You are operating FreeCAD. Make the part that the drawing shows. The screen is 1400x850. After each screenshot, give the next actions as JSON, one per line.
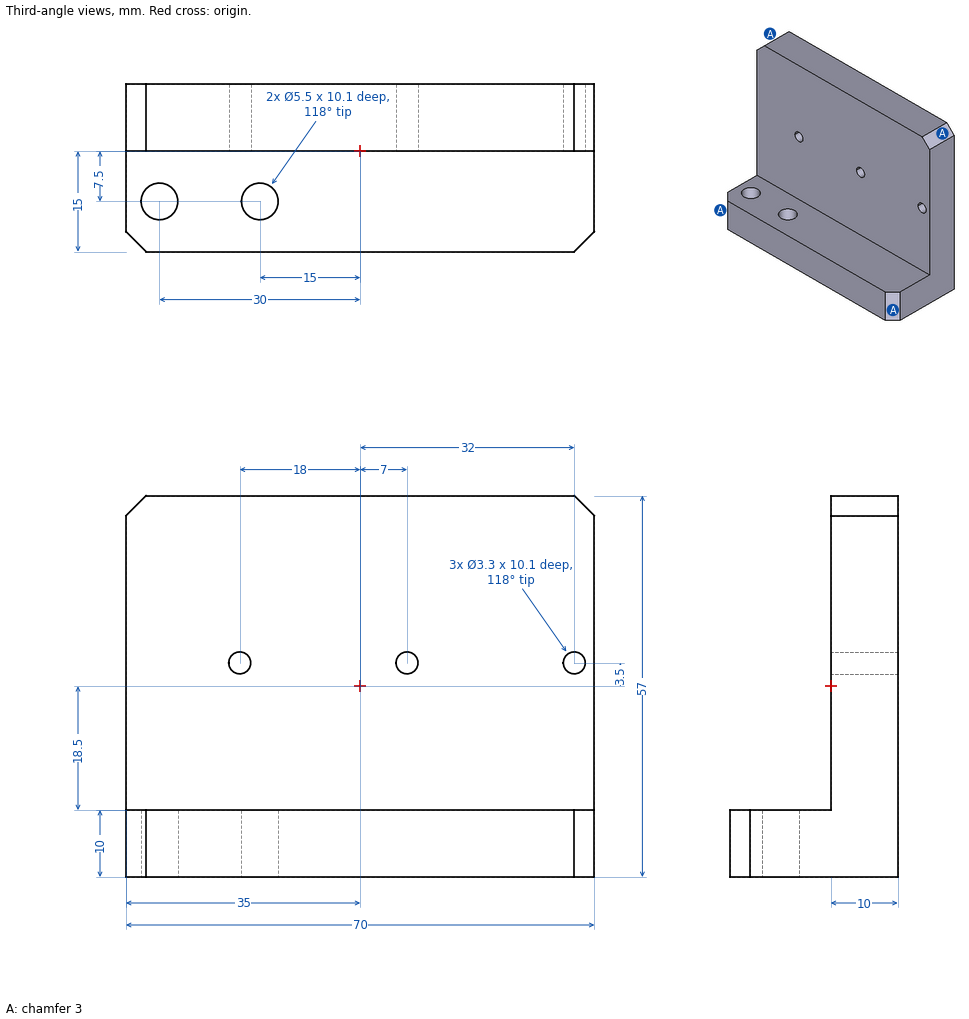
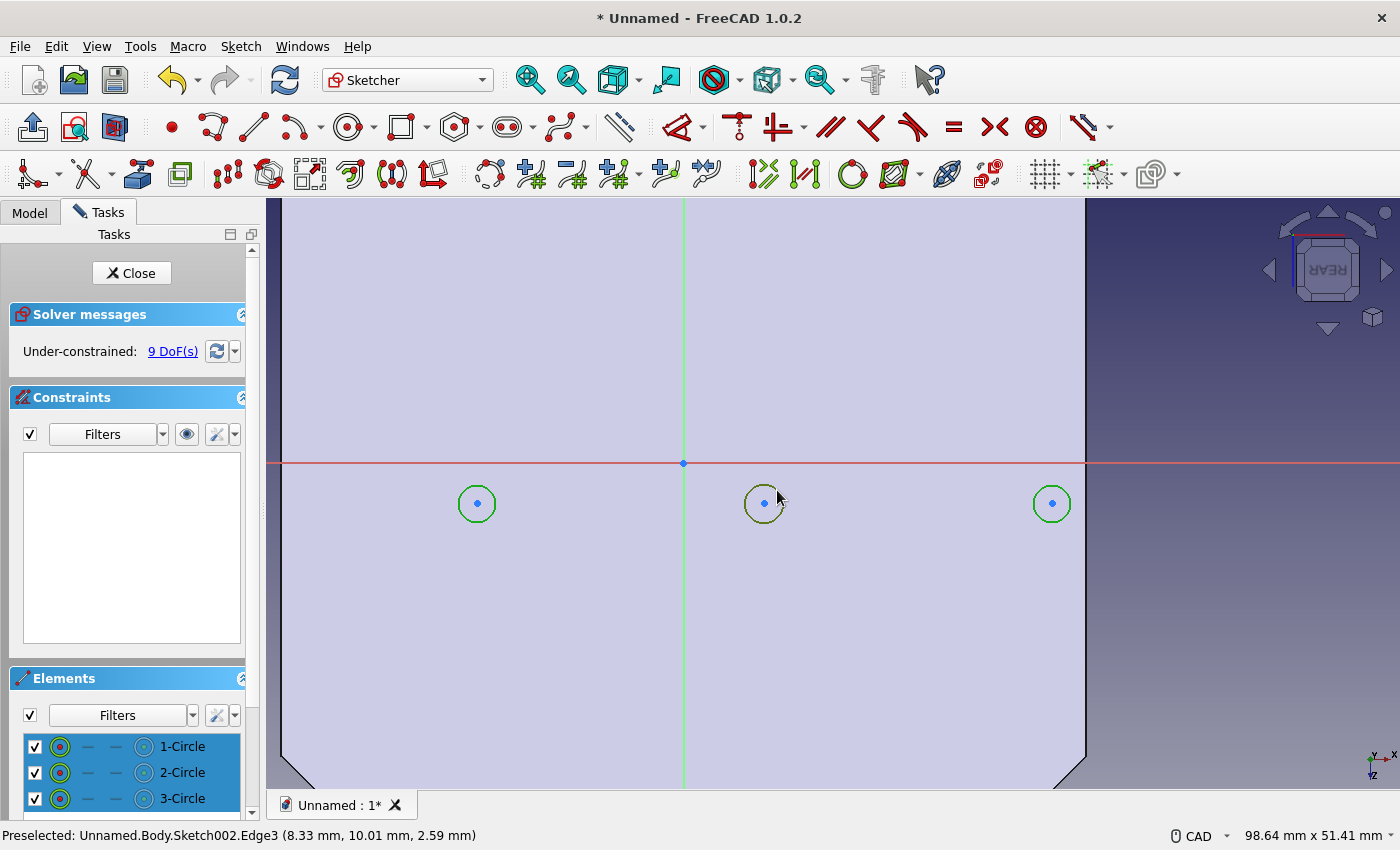
{"action": "left_click", "coordinate": [954, 128]}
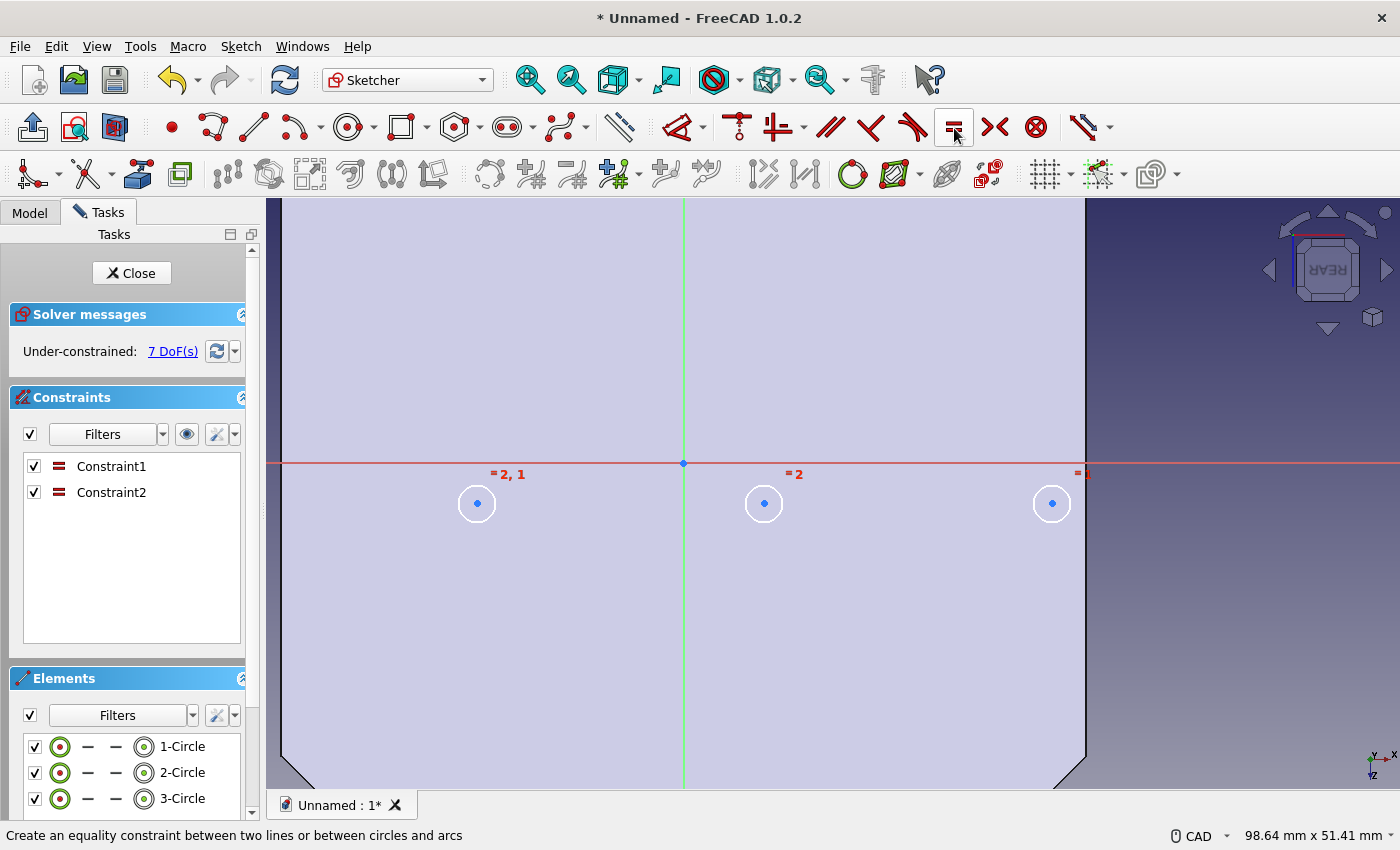
{"action": "left_click", "coordinate": [1052, 504]}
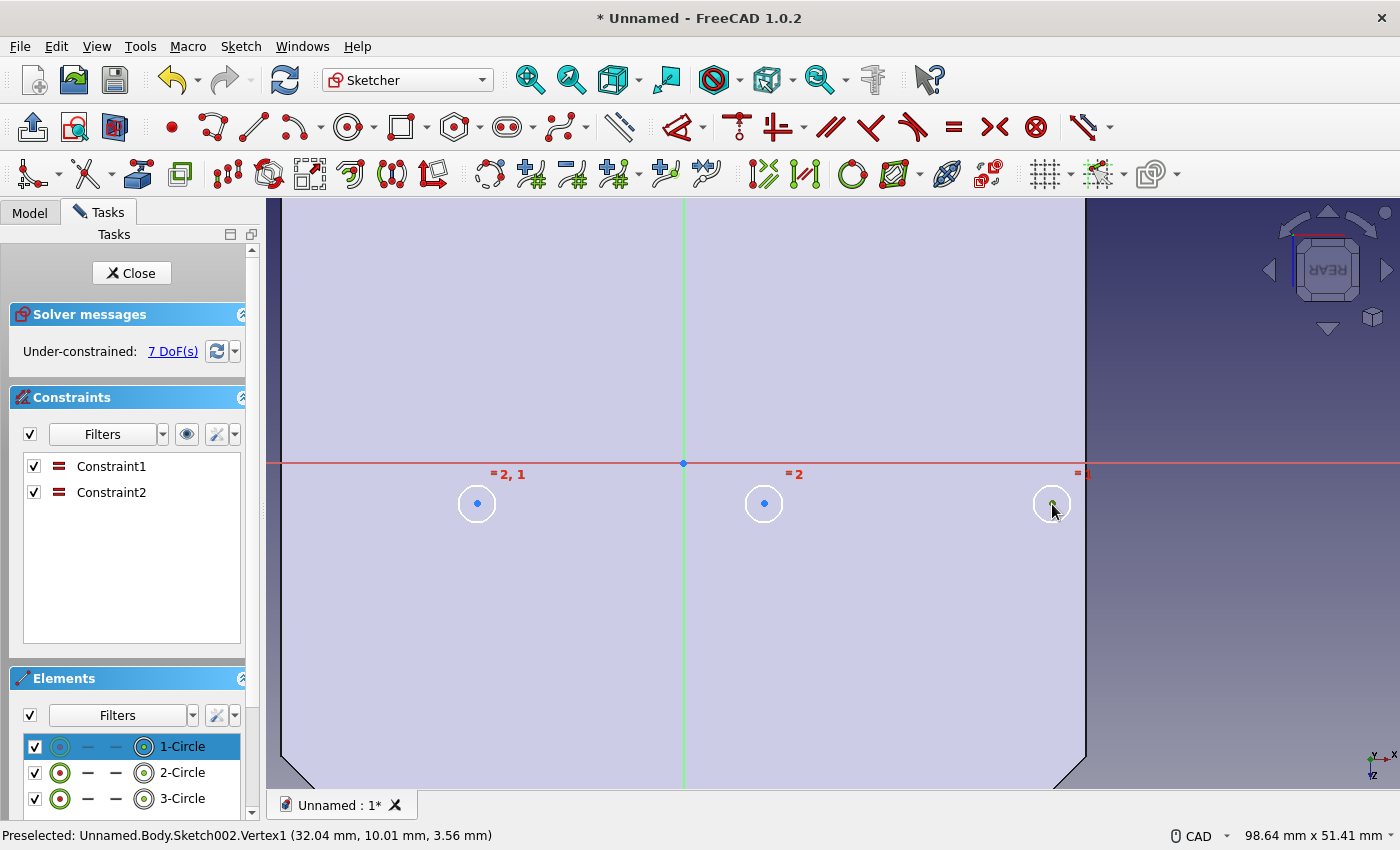
{"action": "left_click", "coordinate": [477, 504]}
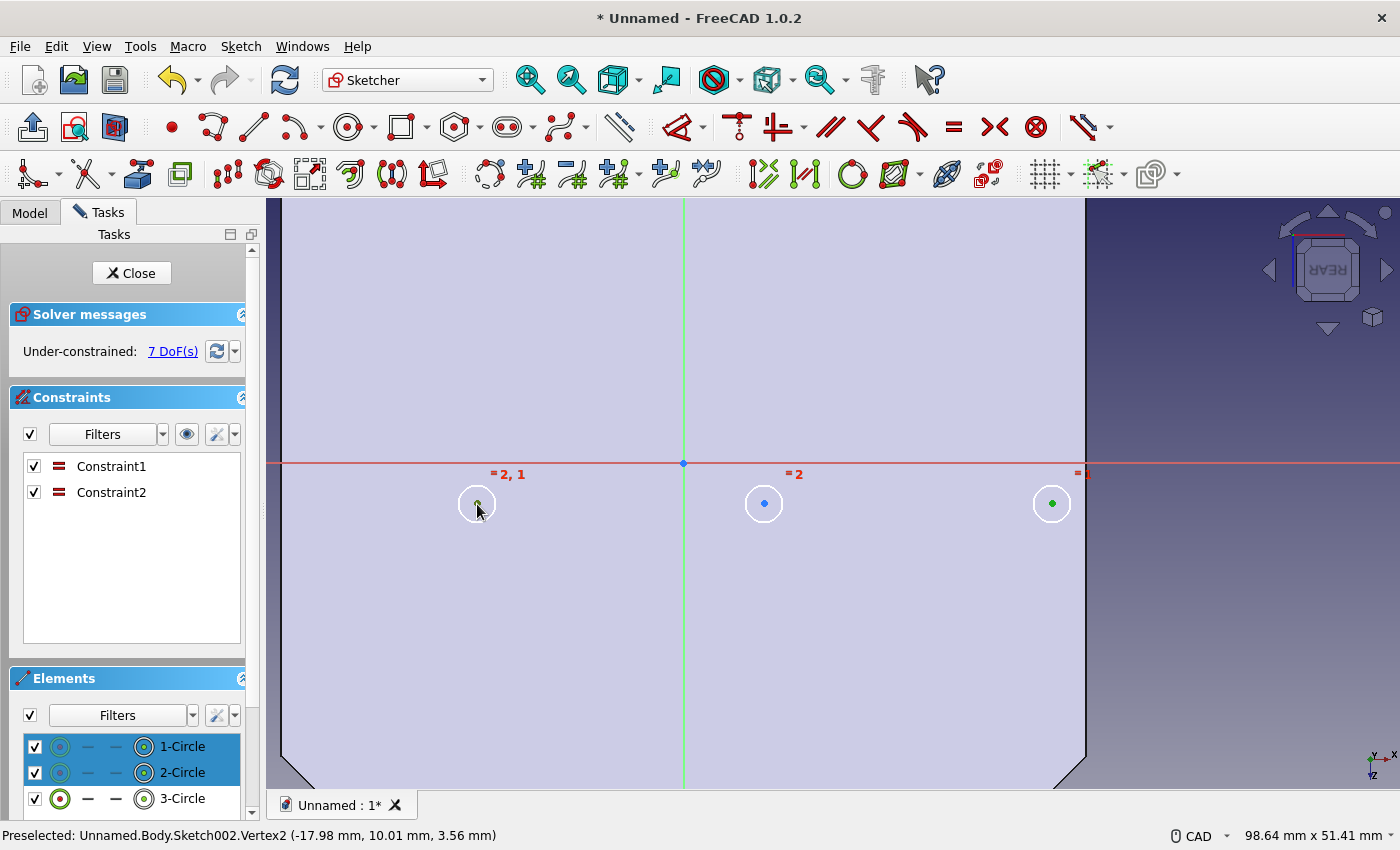
{"action": "left_click", "coordinate": [804, 128]}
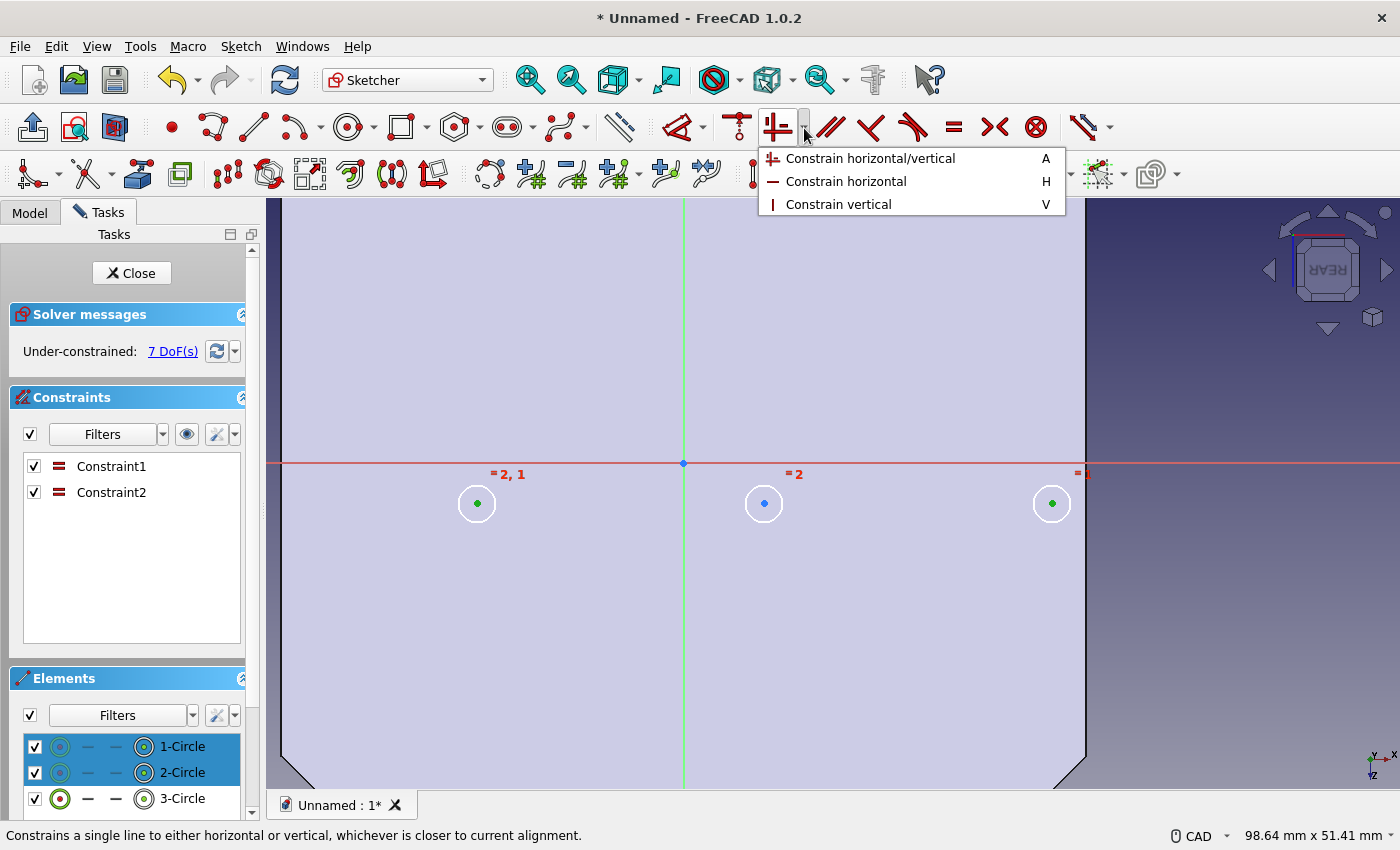
{"action": "left_click", "coordinate": [912, 182]}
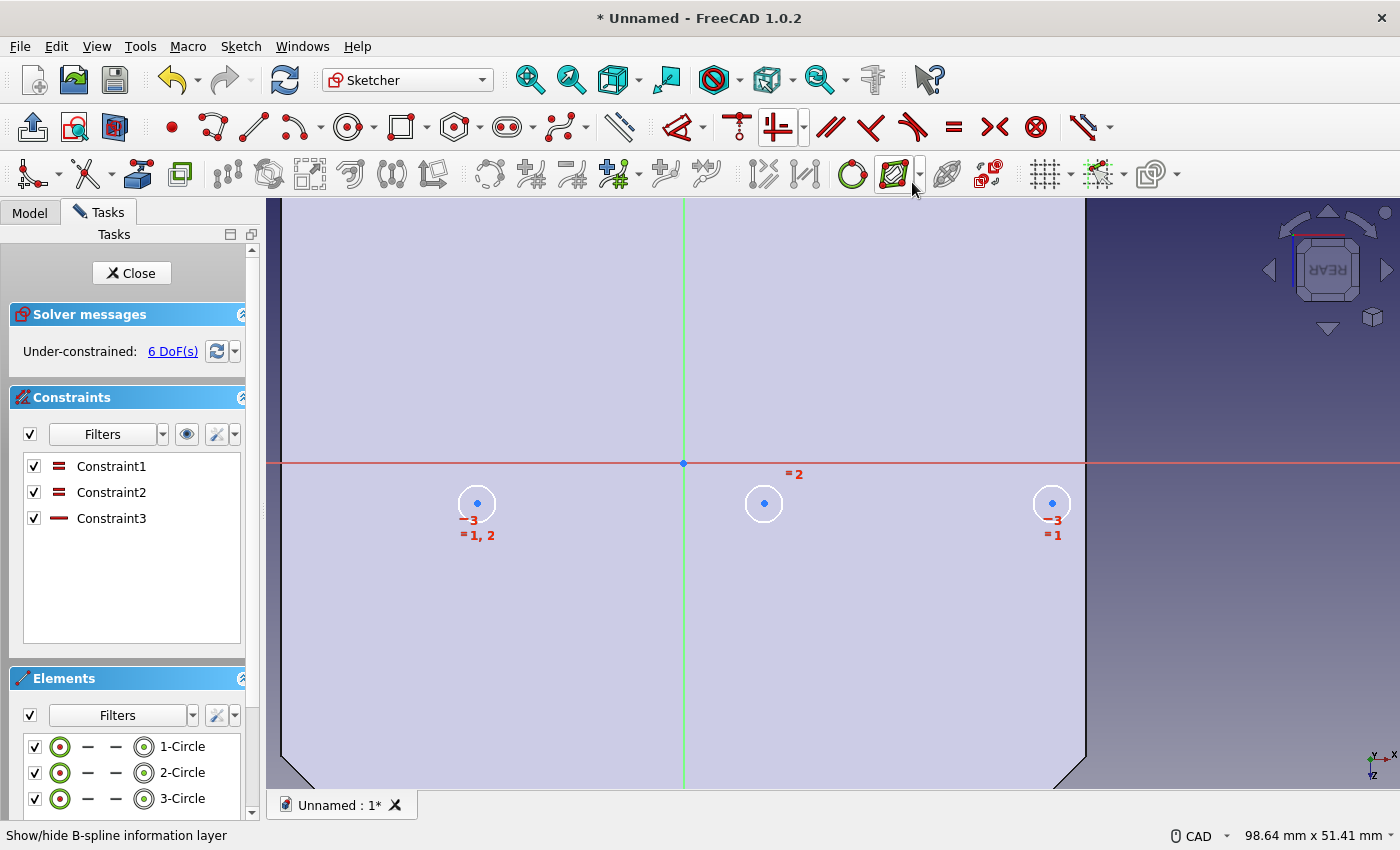
{"action": "left_click", "coordinate": [1052, 504]}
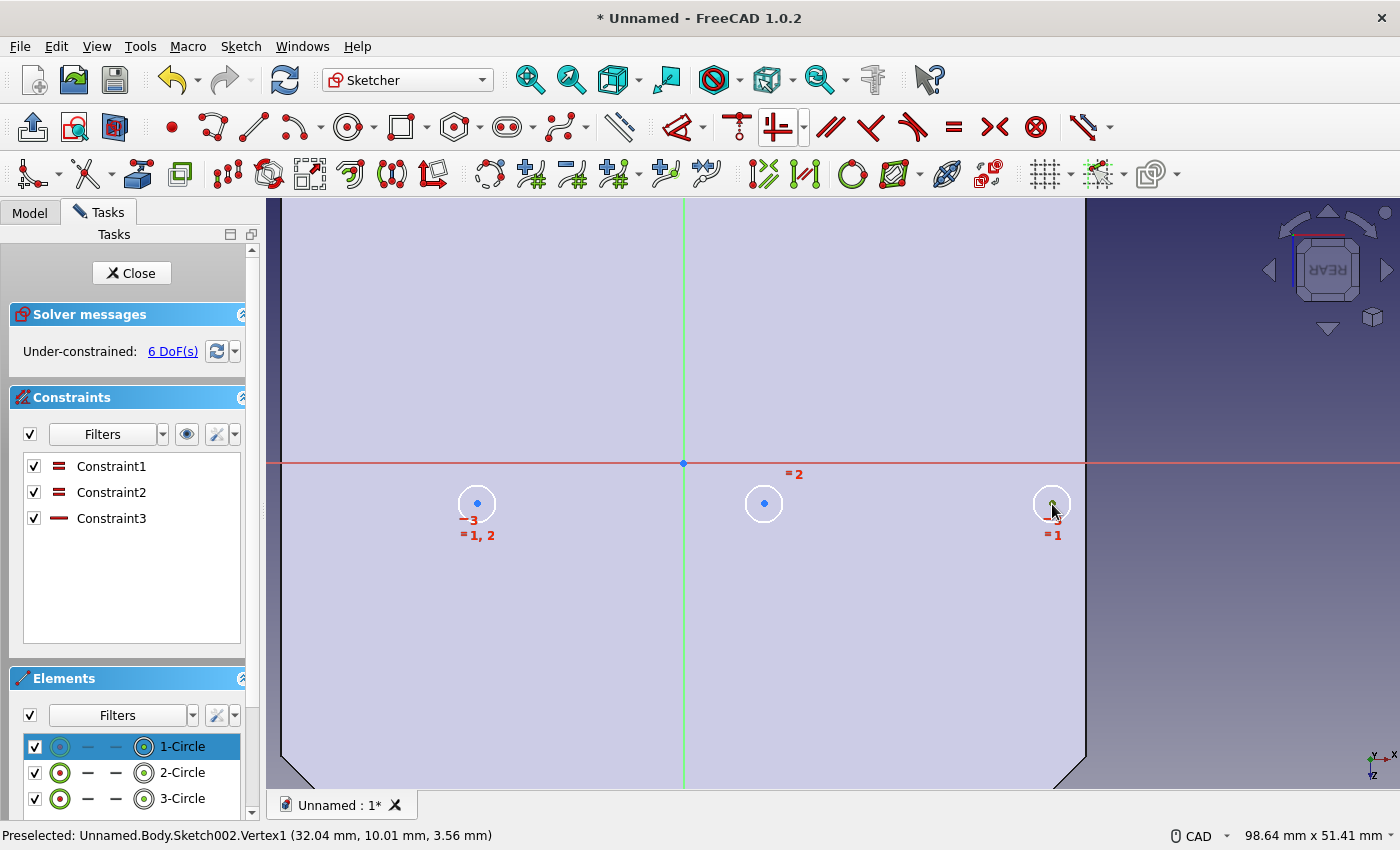
{"action": "left_click", "coordinate": [764, 504]}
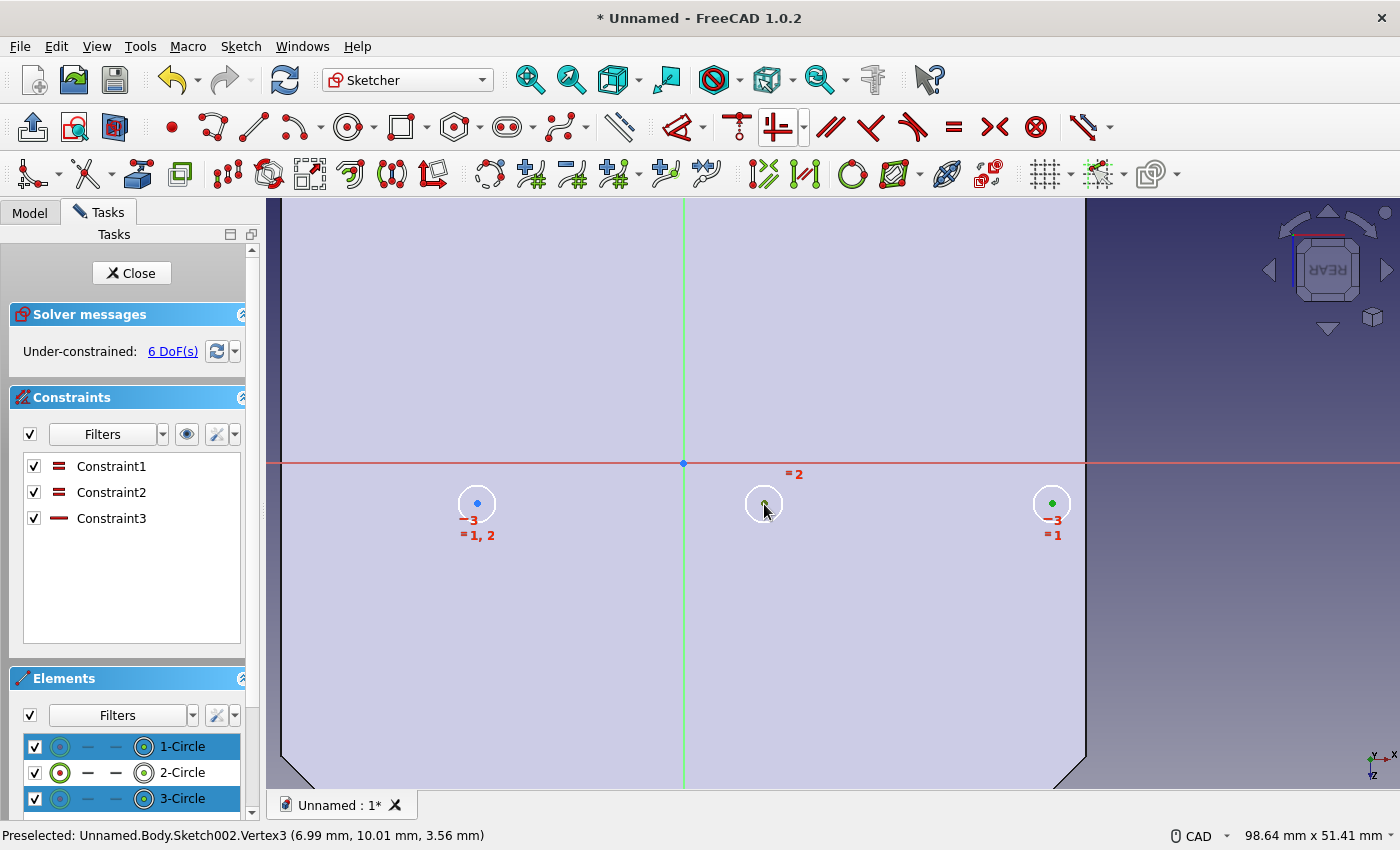
{"action": "key", "text": "h"}